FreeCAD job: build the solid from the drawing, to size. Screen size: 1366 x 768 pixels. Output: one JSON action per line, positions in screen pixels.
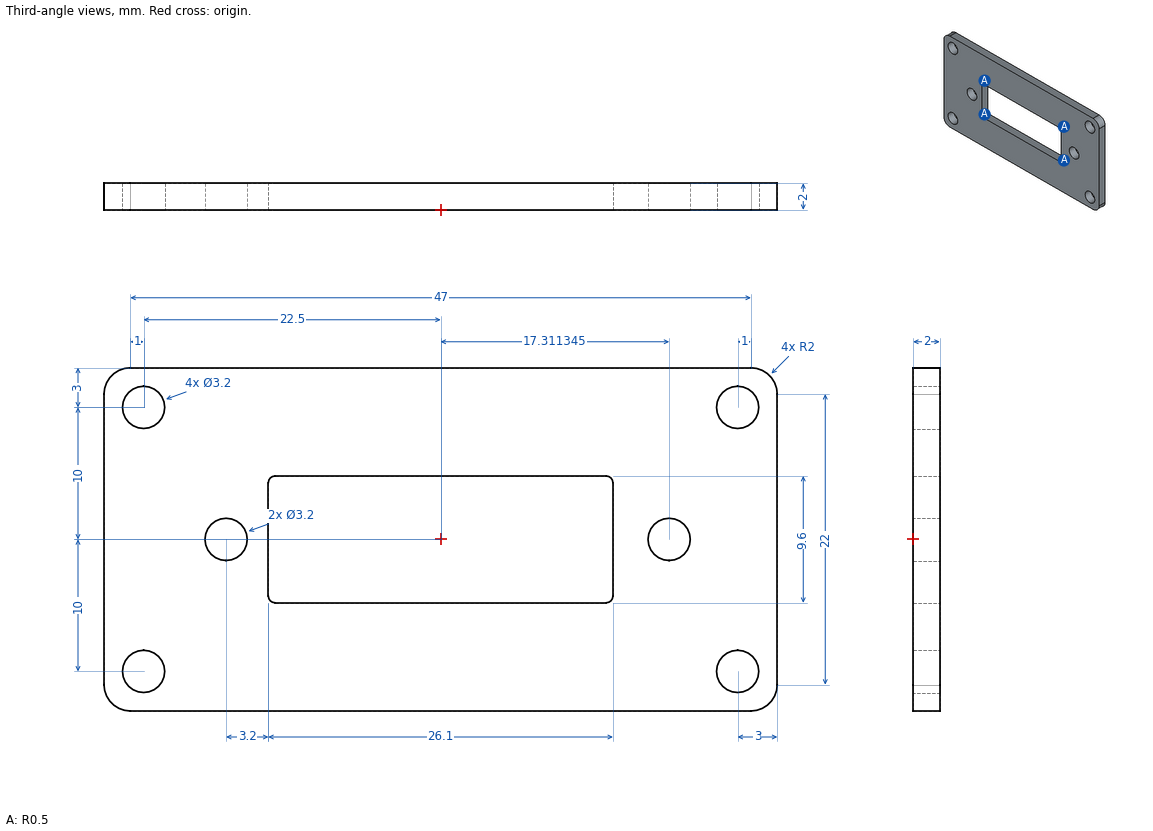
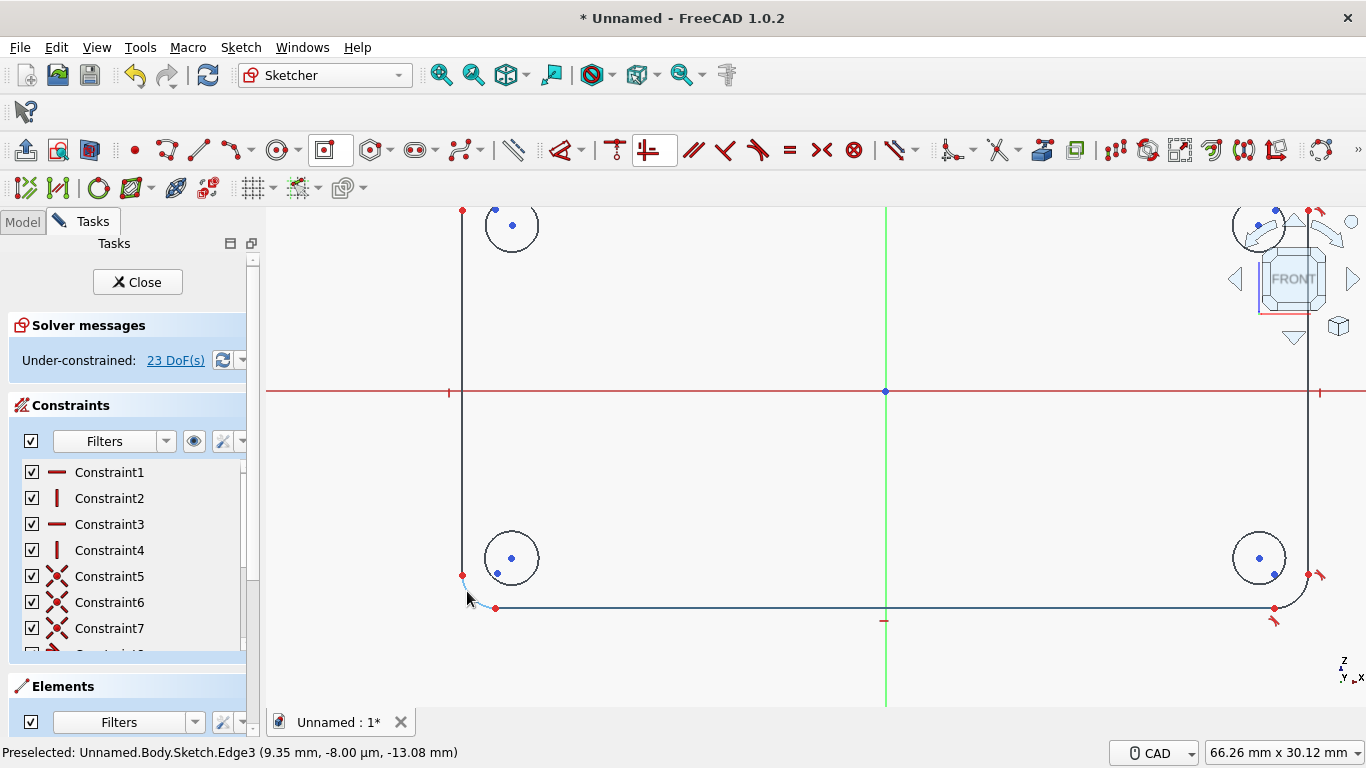
{"action": "left_click", "coordinate": [467, 590]}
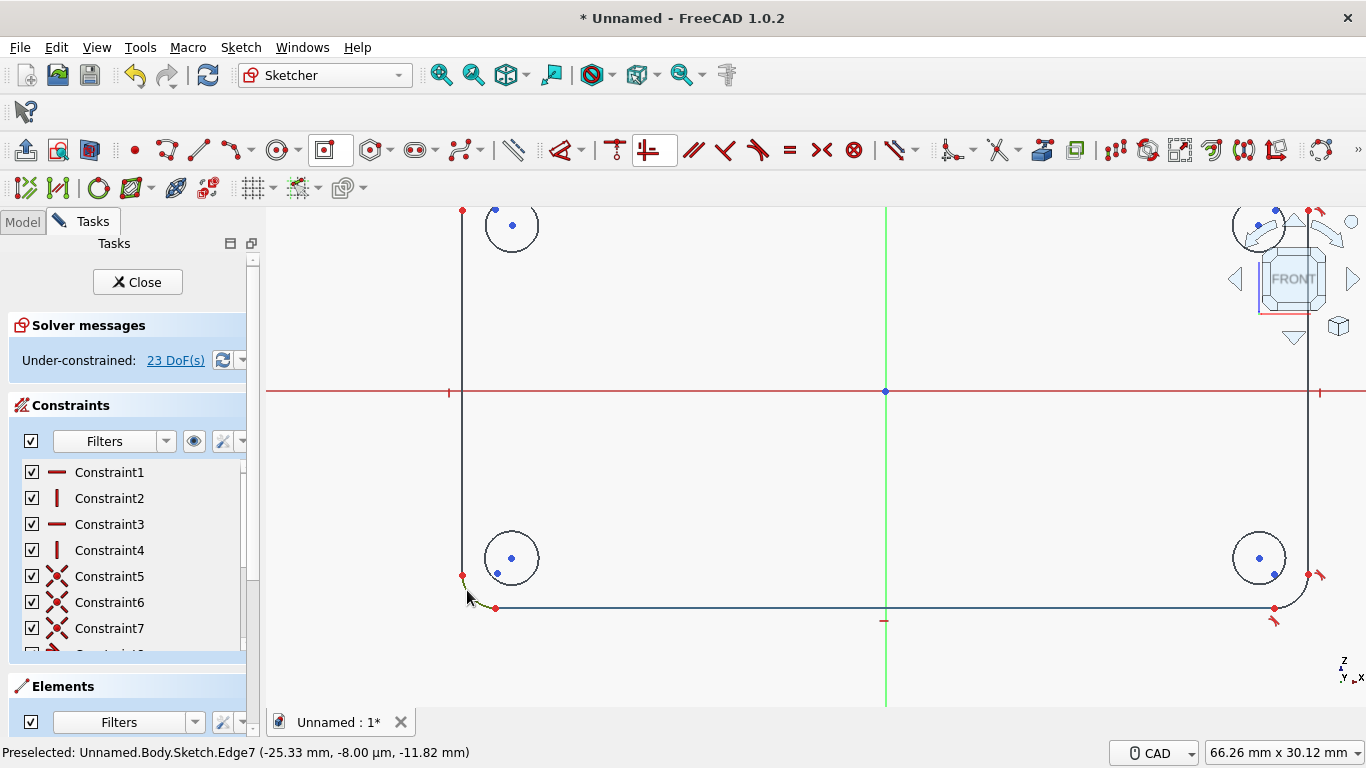
{"action": "left_click", "coordinate": [758, 150]}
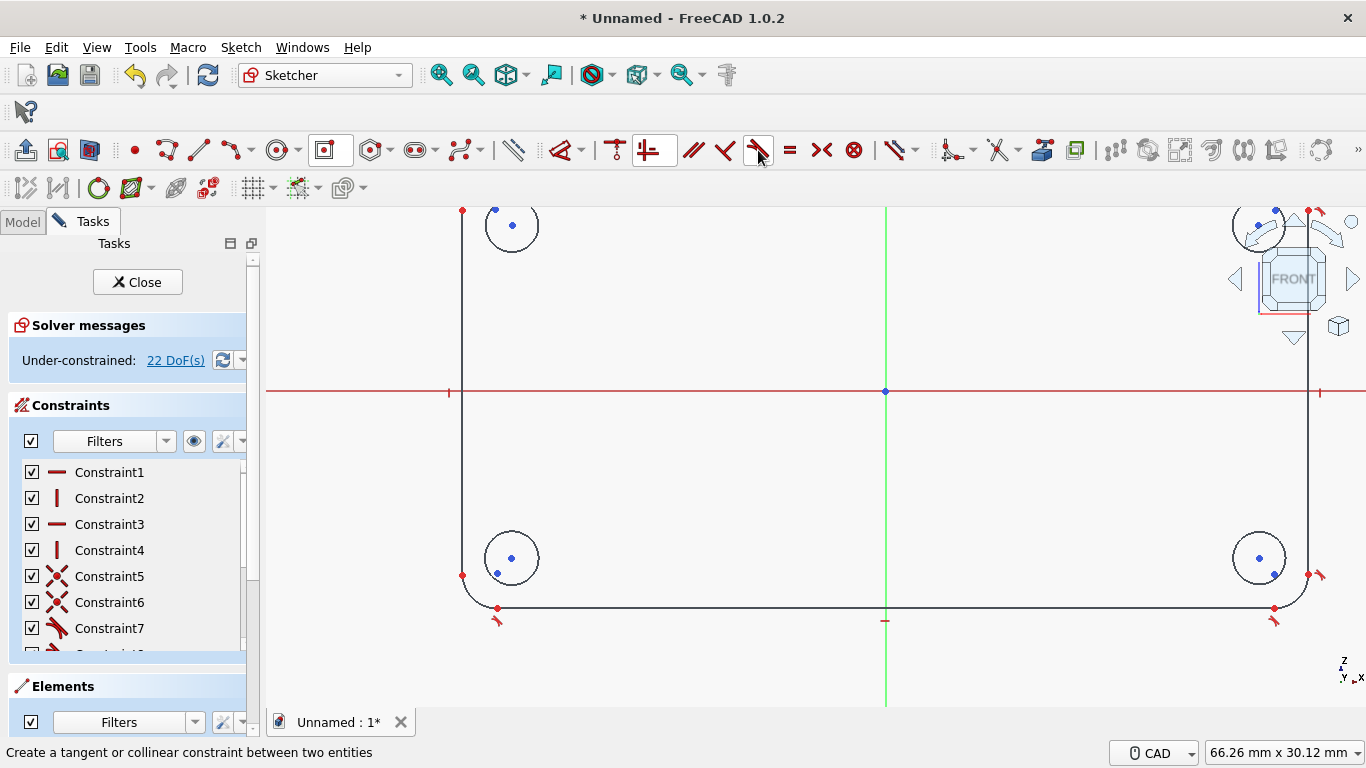
{"action": "left_click", "coordinate": [462, 466]}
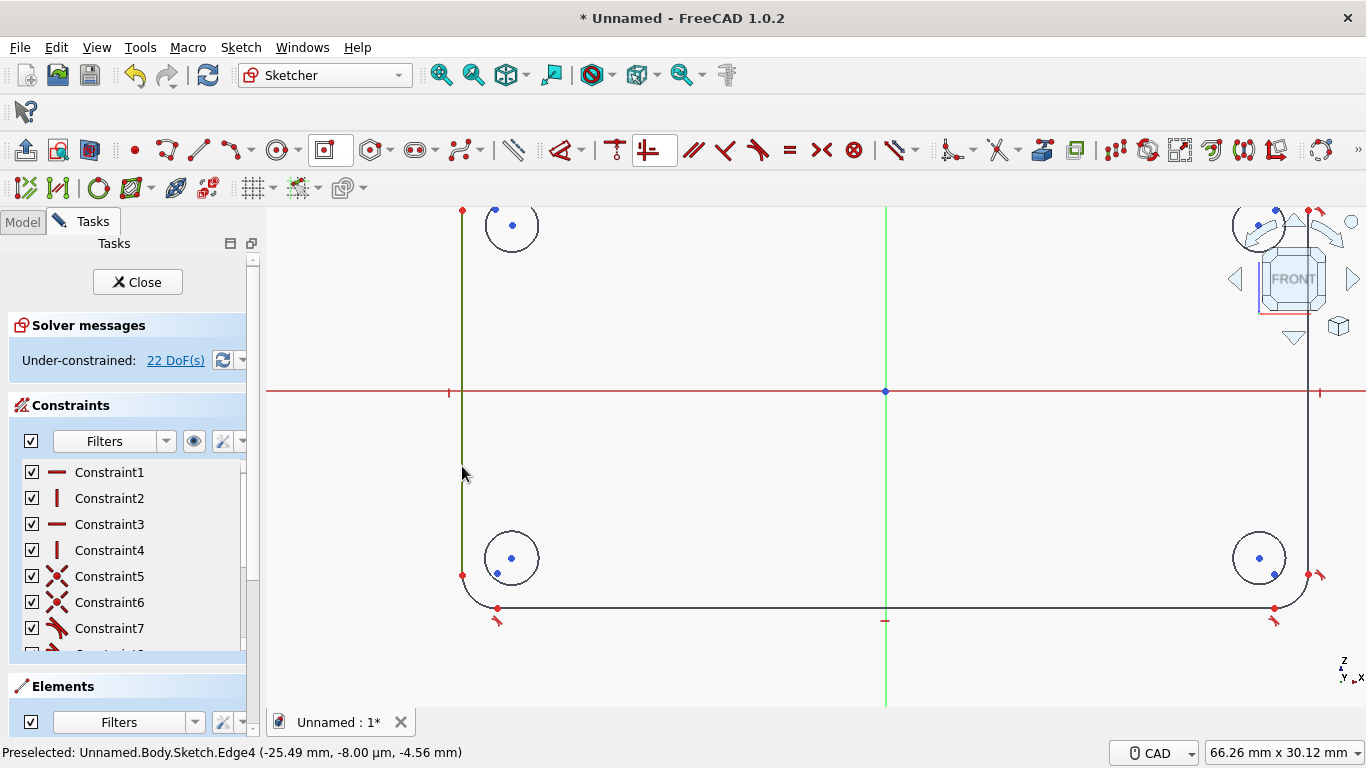
{"action": "left_click", "coordinate": [467, 591]}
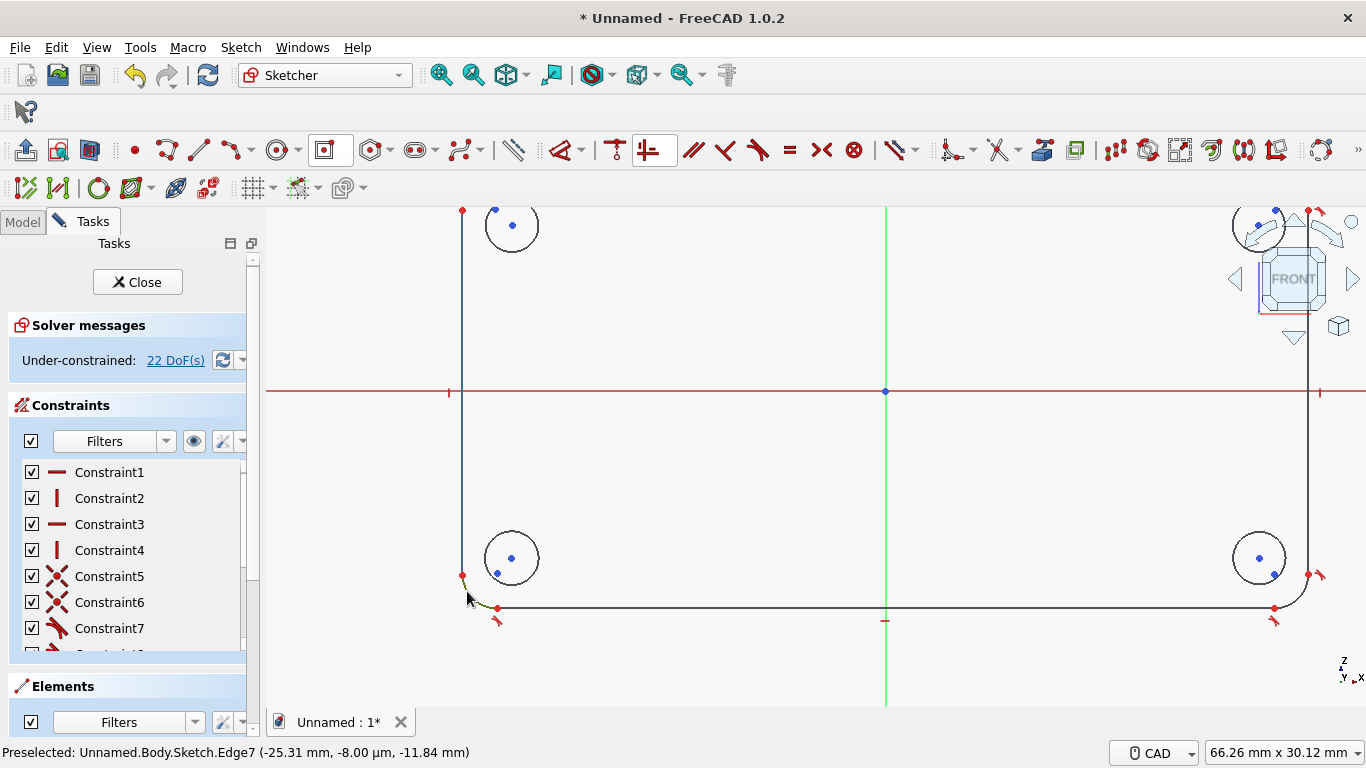
{"action": "left_click", "coordinate": [758, 150]}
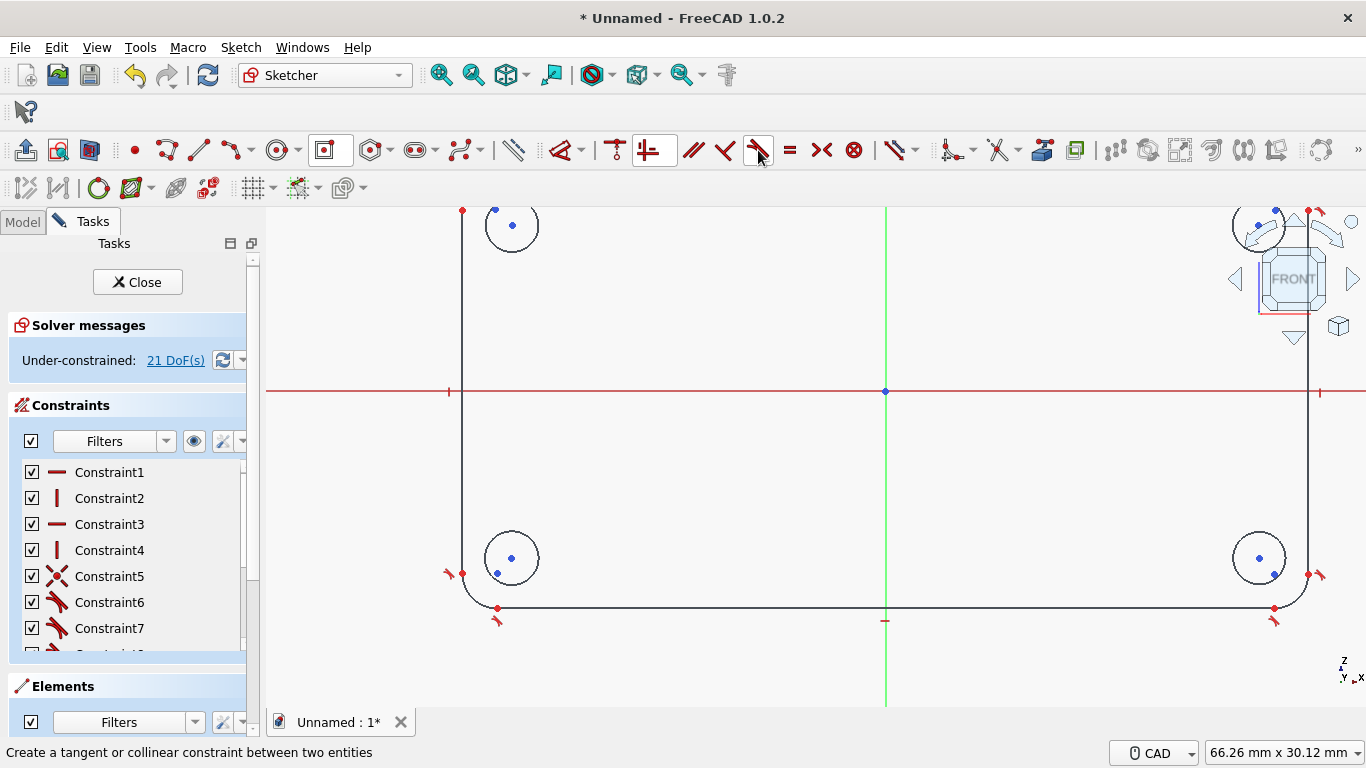
{"action": "left_click", "coordinate": [462, 465]}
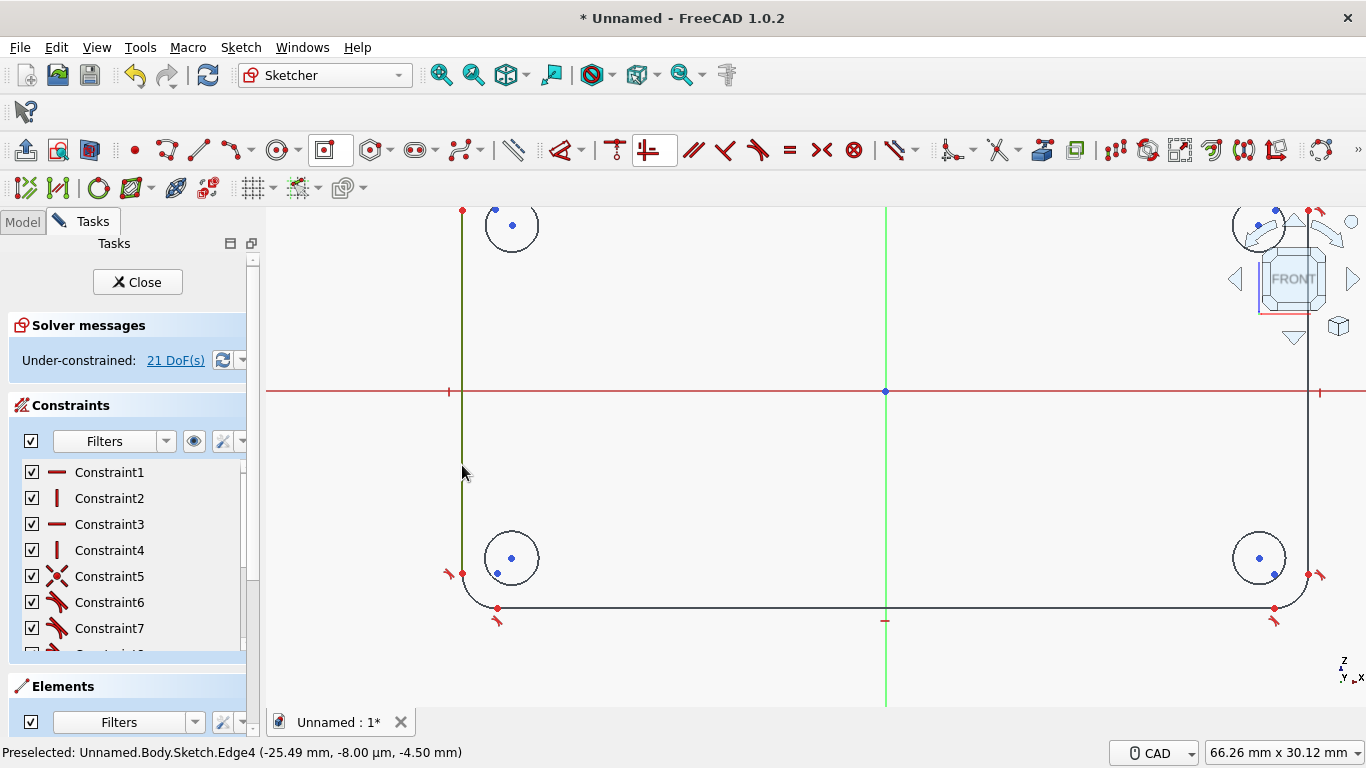
{"action": "scroll", "coordinate": [467, 591], "scroll_direction": "down", "scroll_amount": 2}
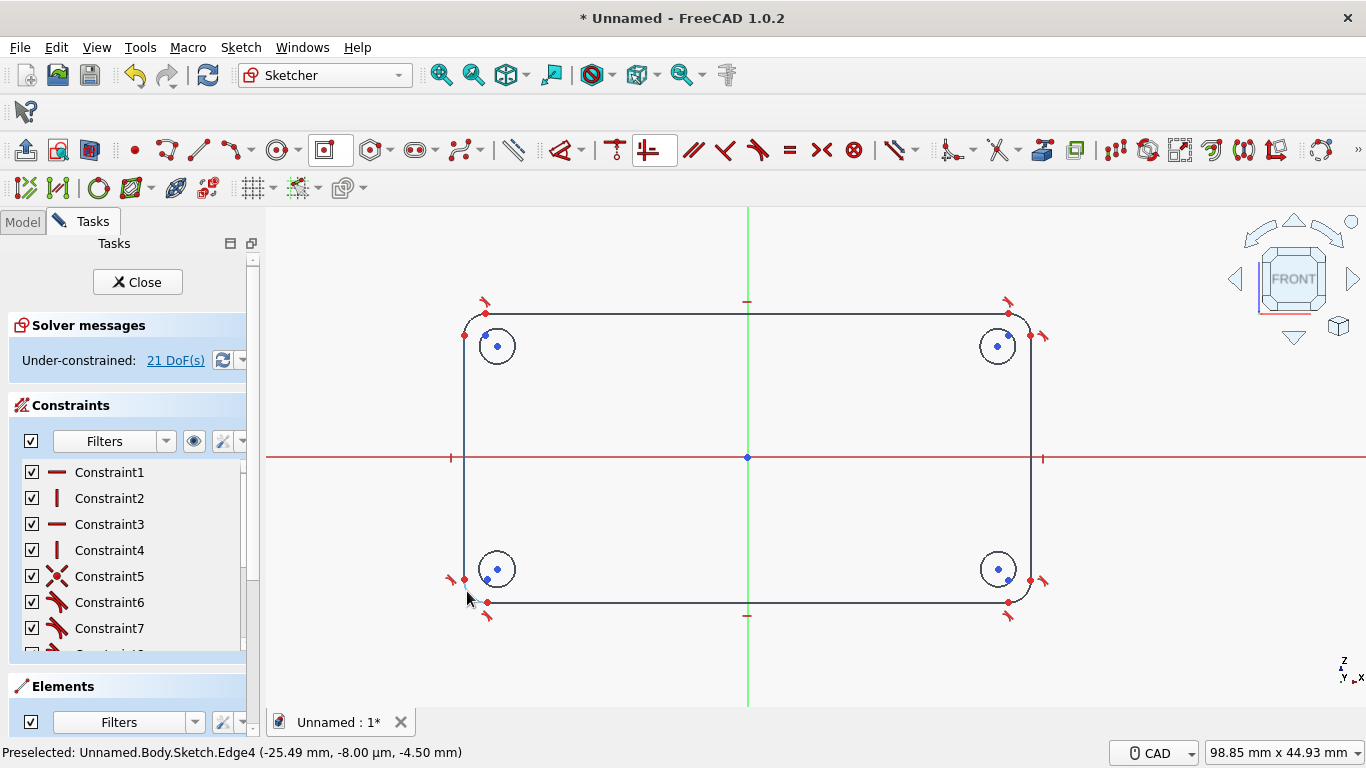
{"action": "scroll", "coordinate": [476, 316], "scroll_direction": "up", "scroll_amount": 2}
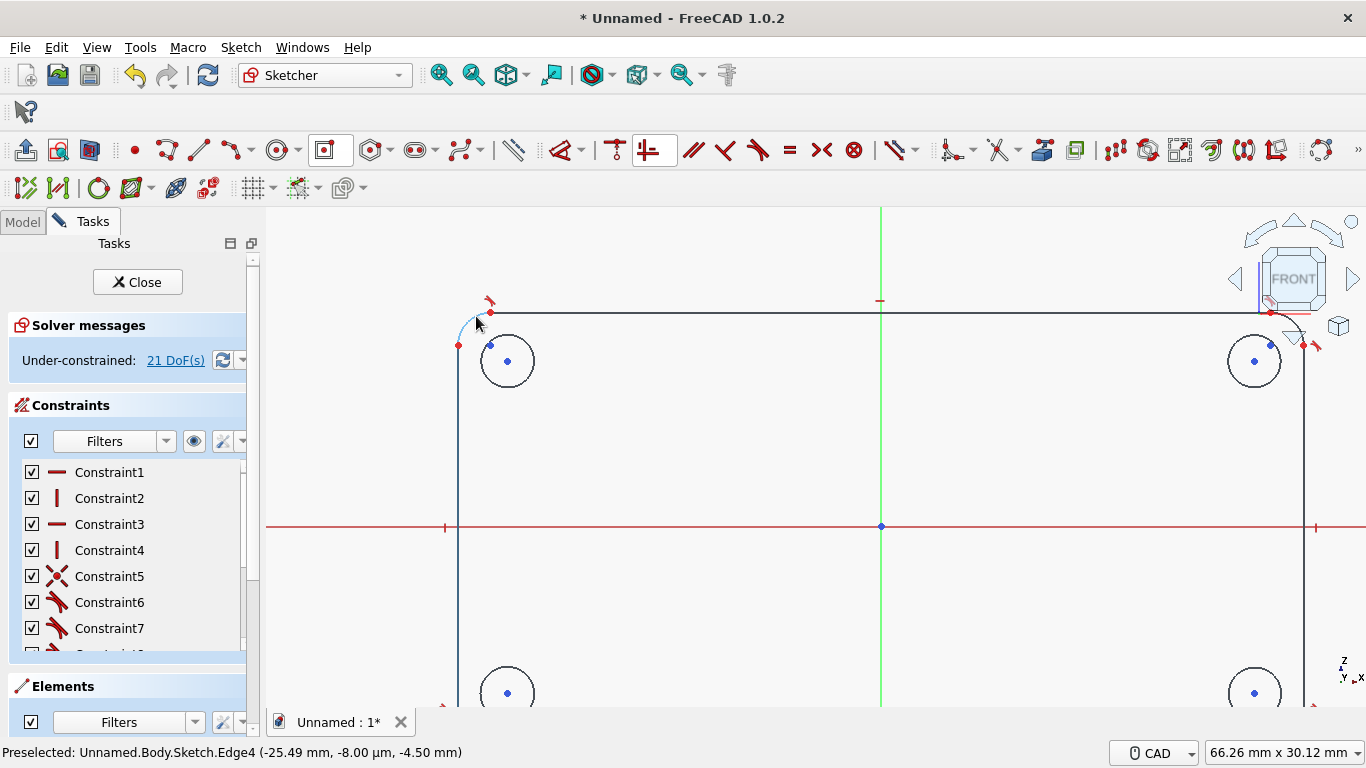
{"action": "left_click", "coordinate": [476, 316]}